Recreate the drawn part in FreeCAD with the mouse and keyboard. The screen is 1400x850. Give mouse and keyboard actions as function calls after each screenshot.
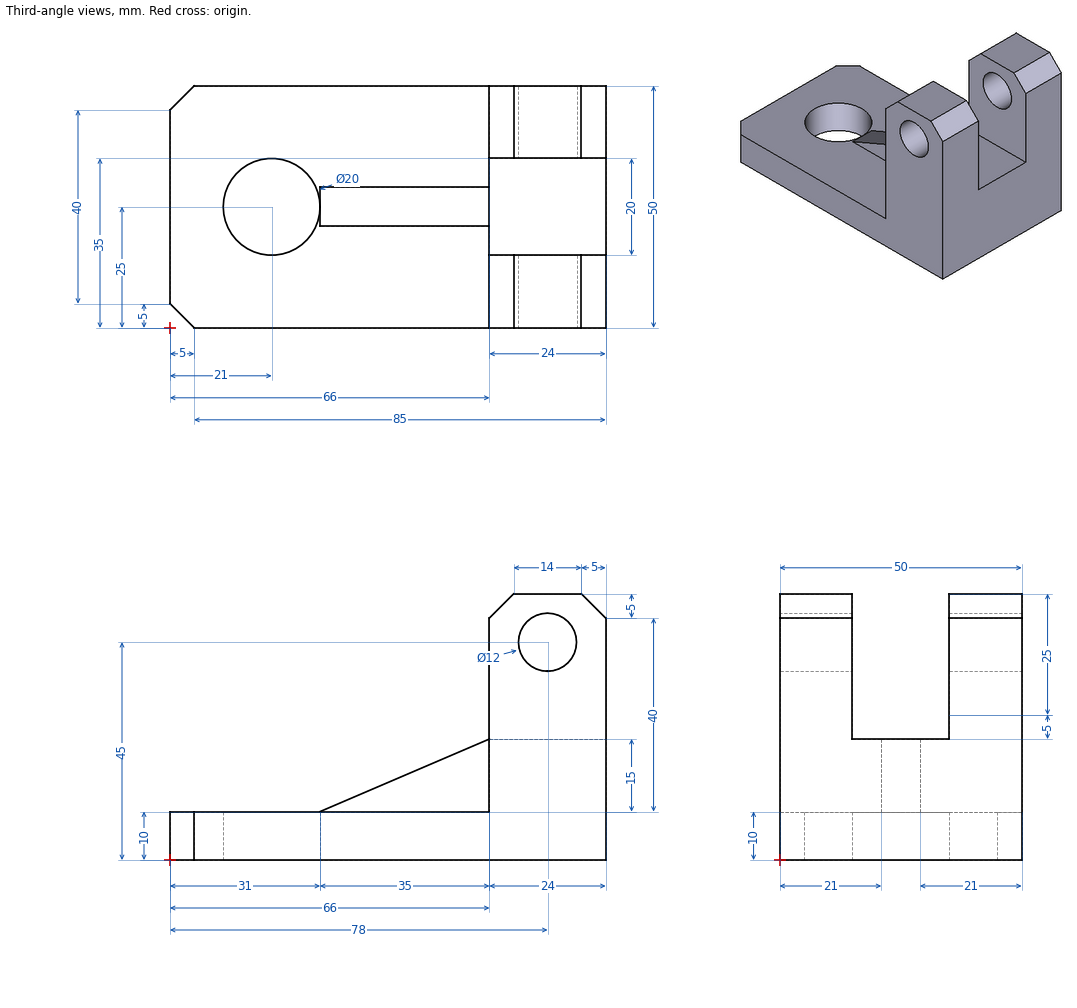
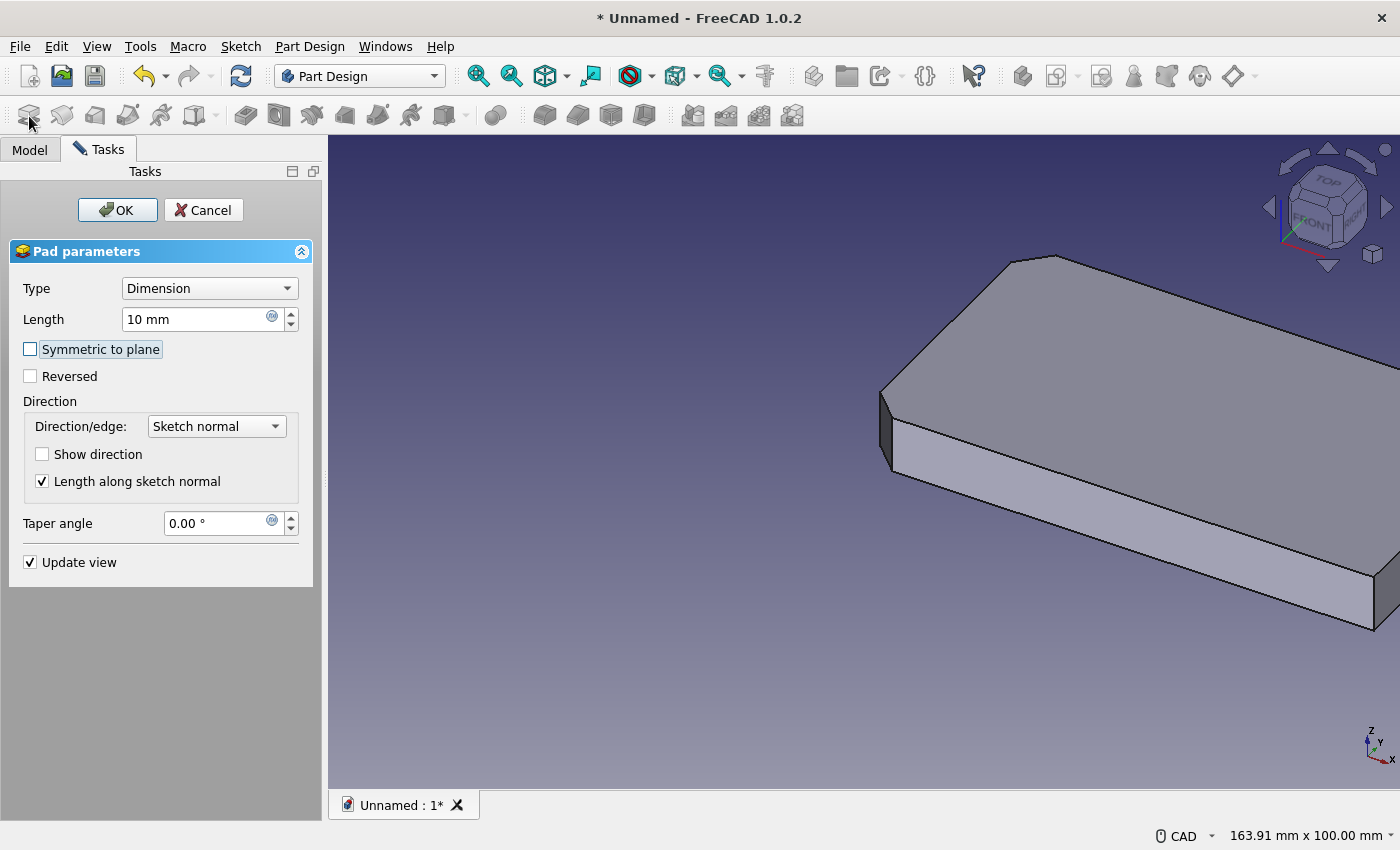
click(118, 210)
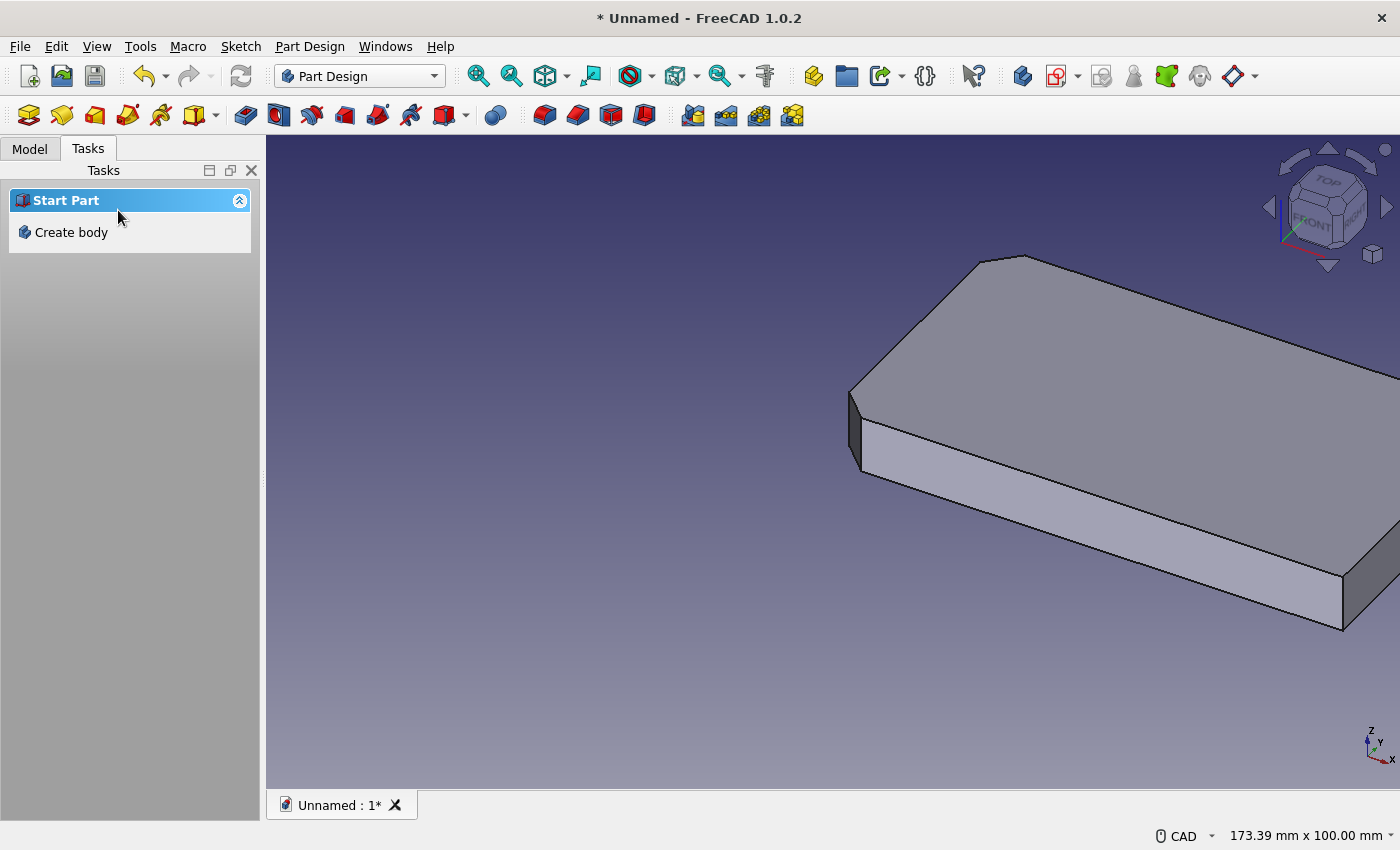
click(479, 76)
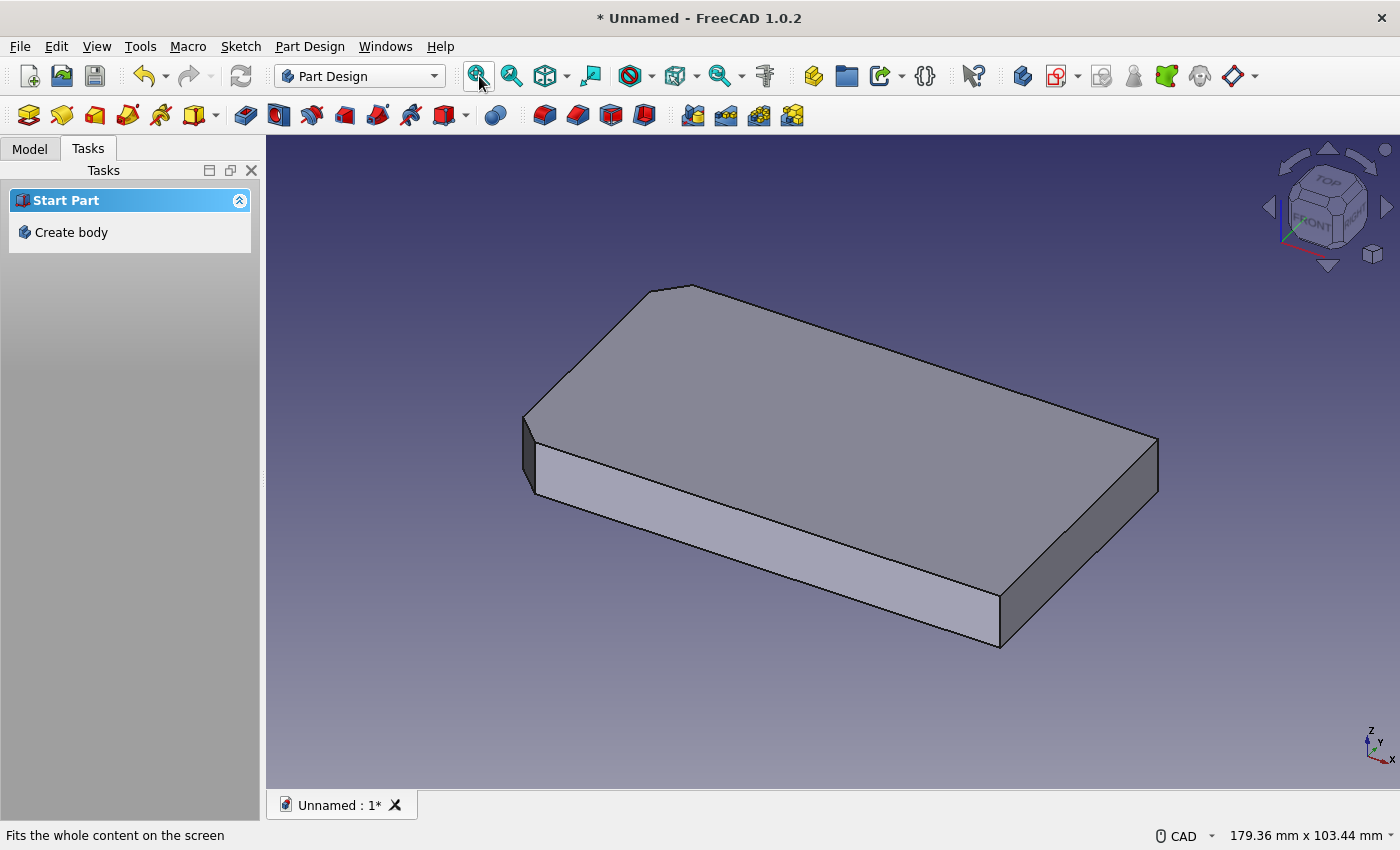
click(967, 610)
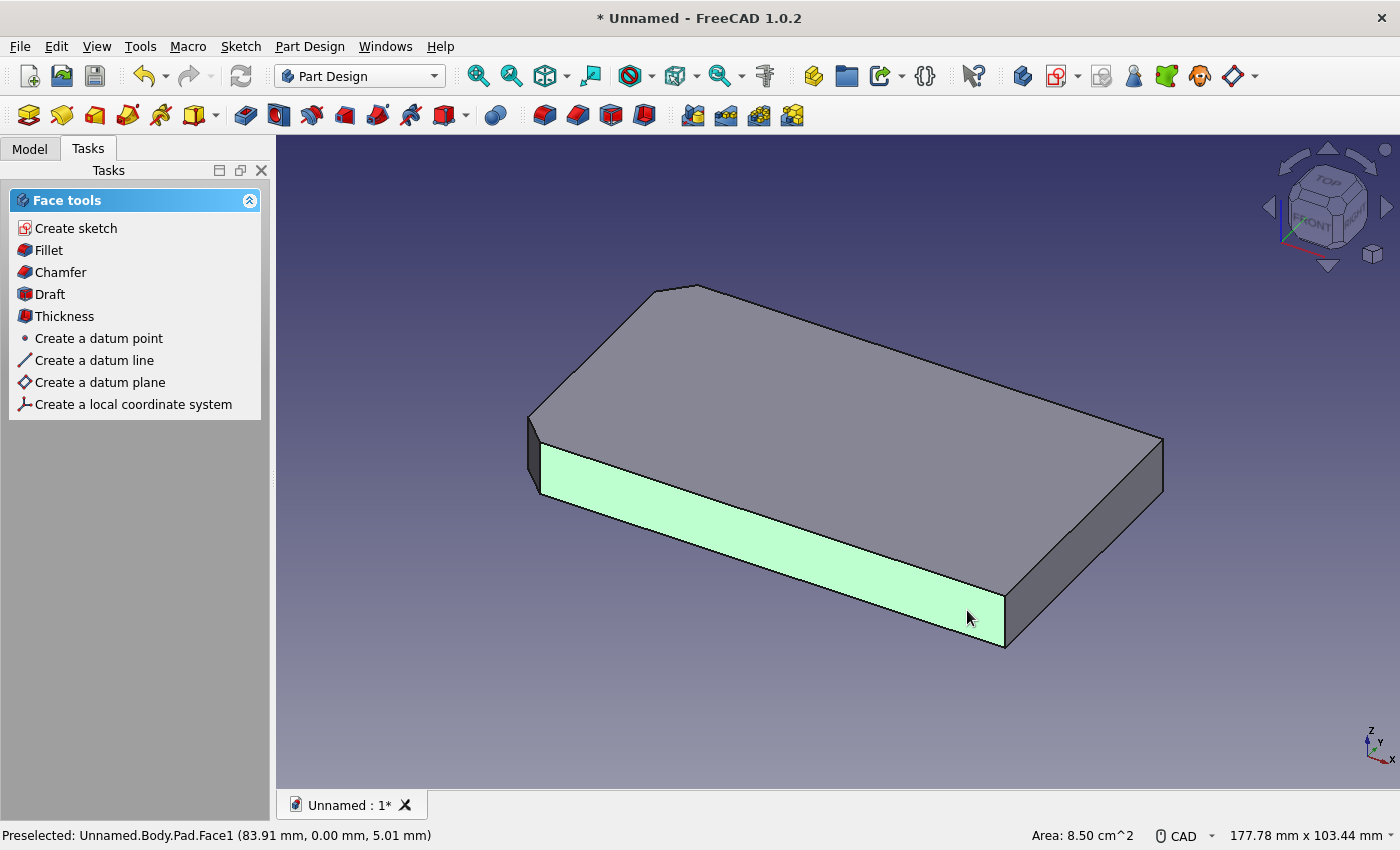
click(1056, 76)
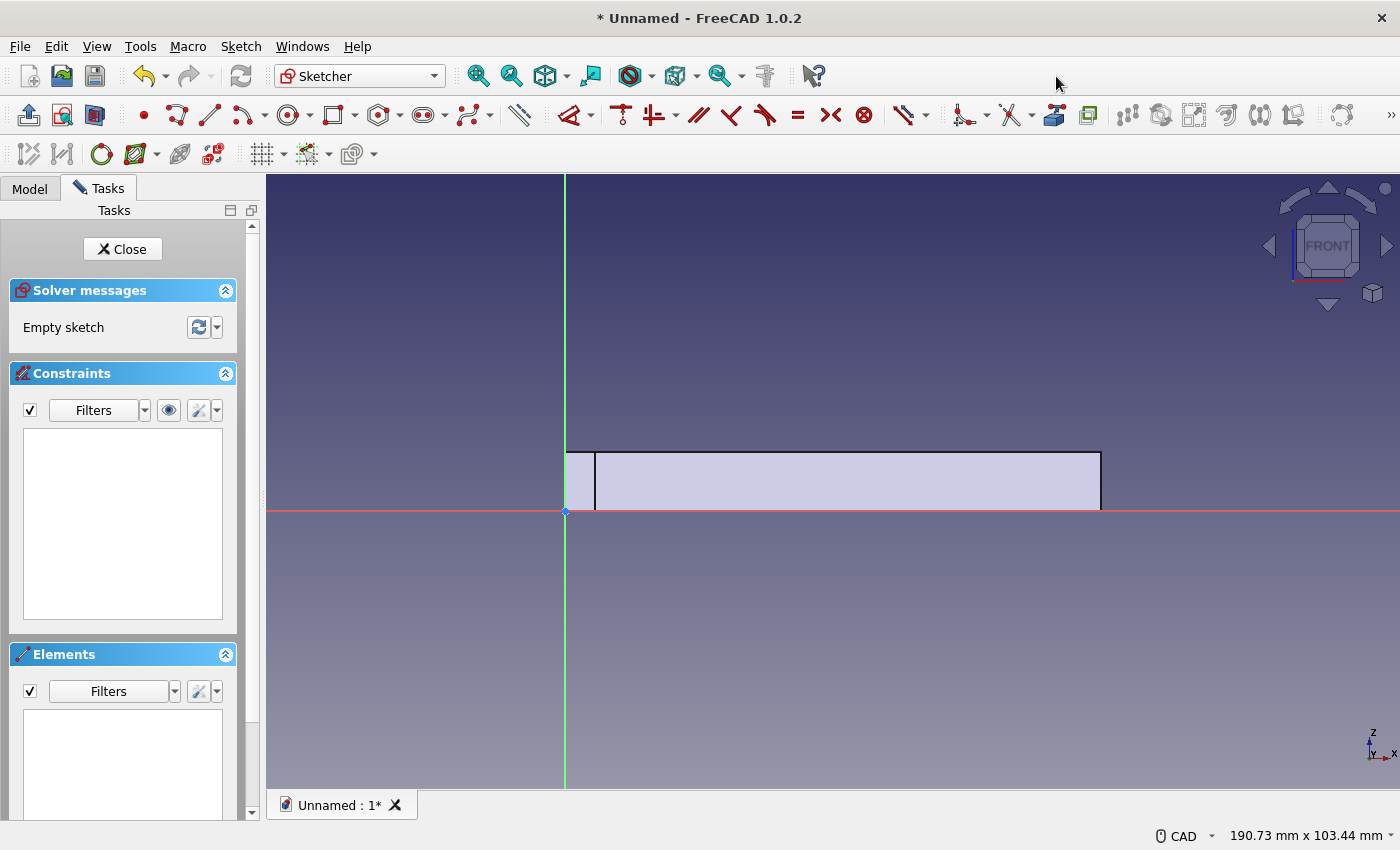
scroll(455, 761, down, 1)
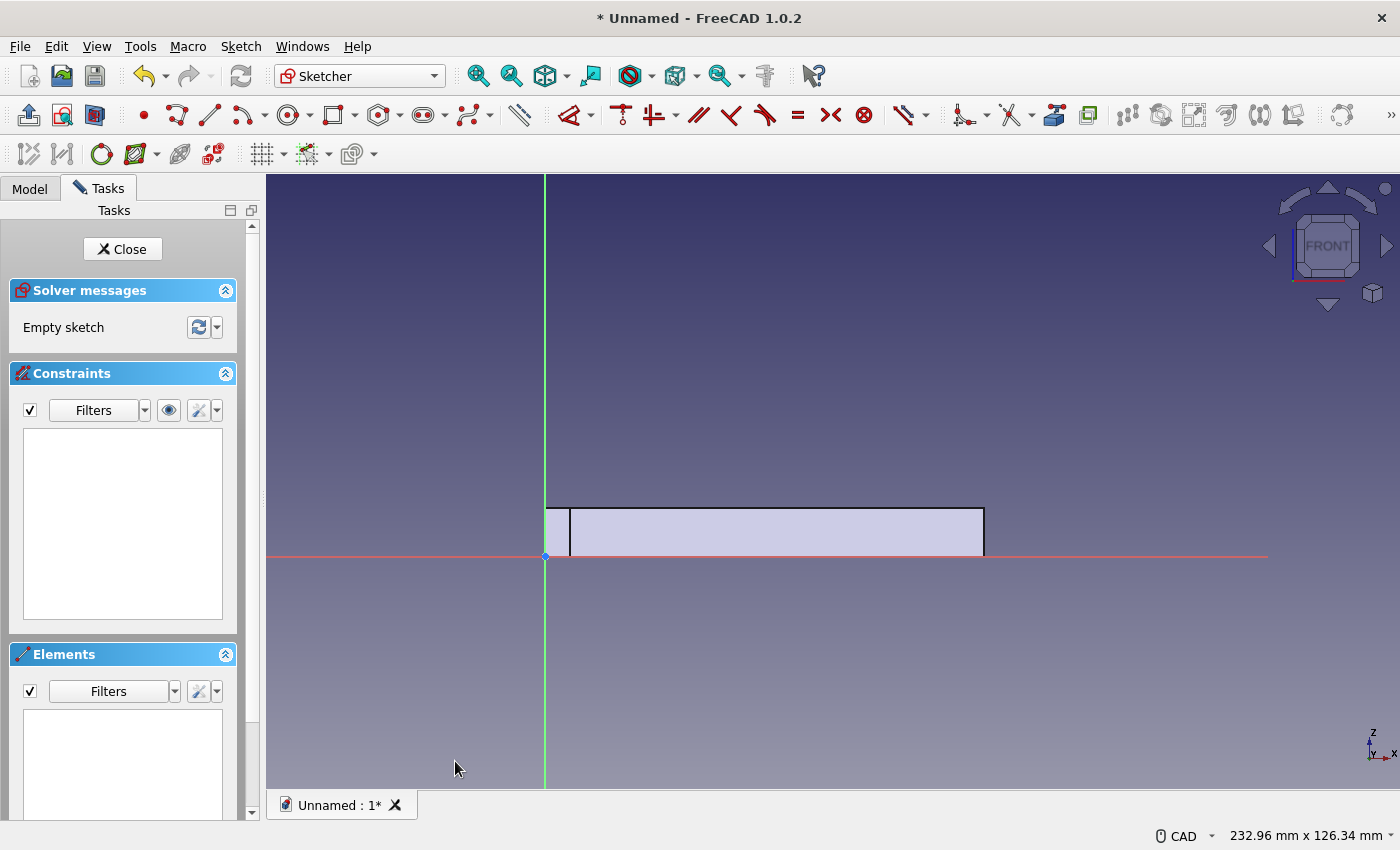
scroll(765, 303, up, 2)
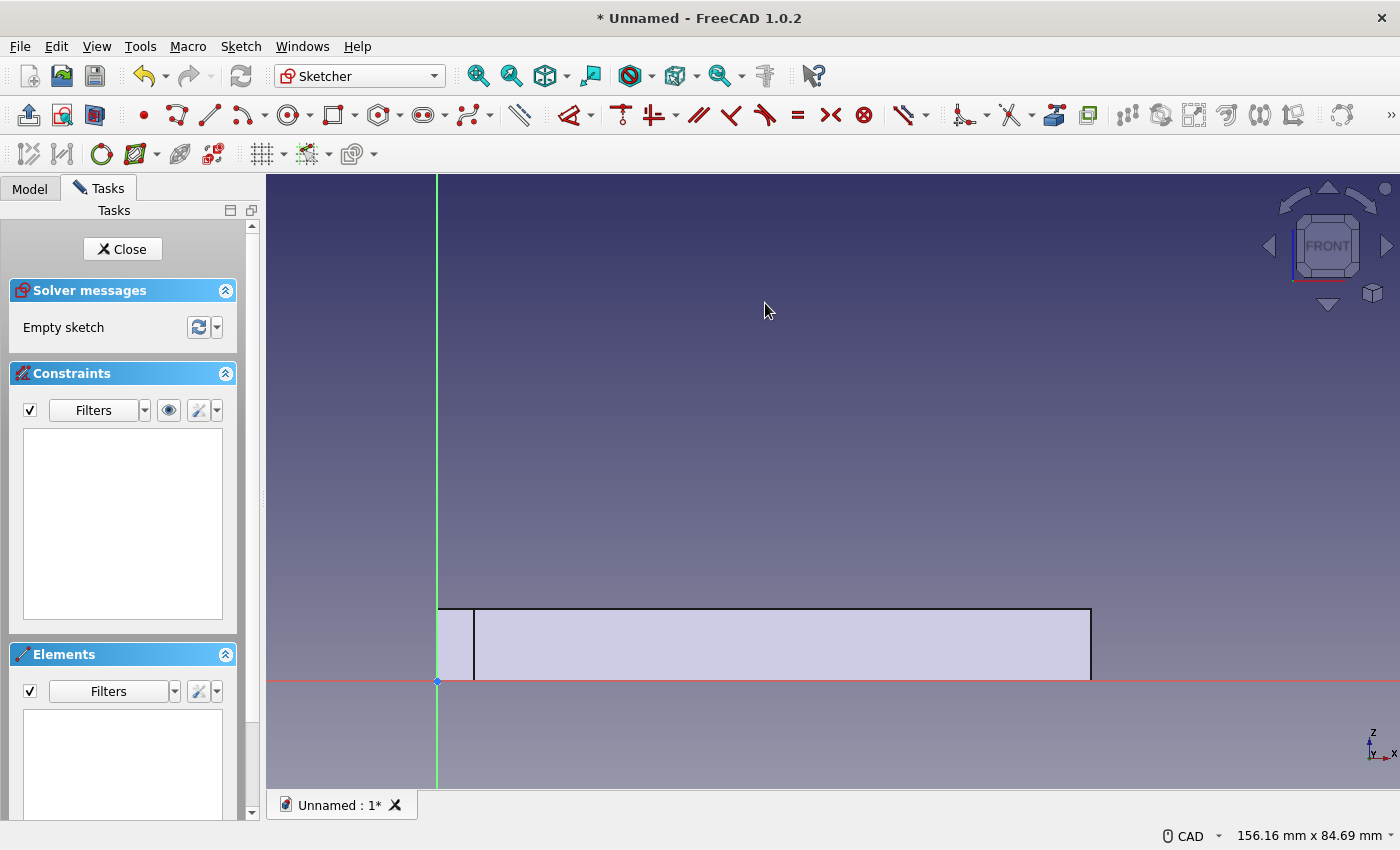
click(177, 116)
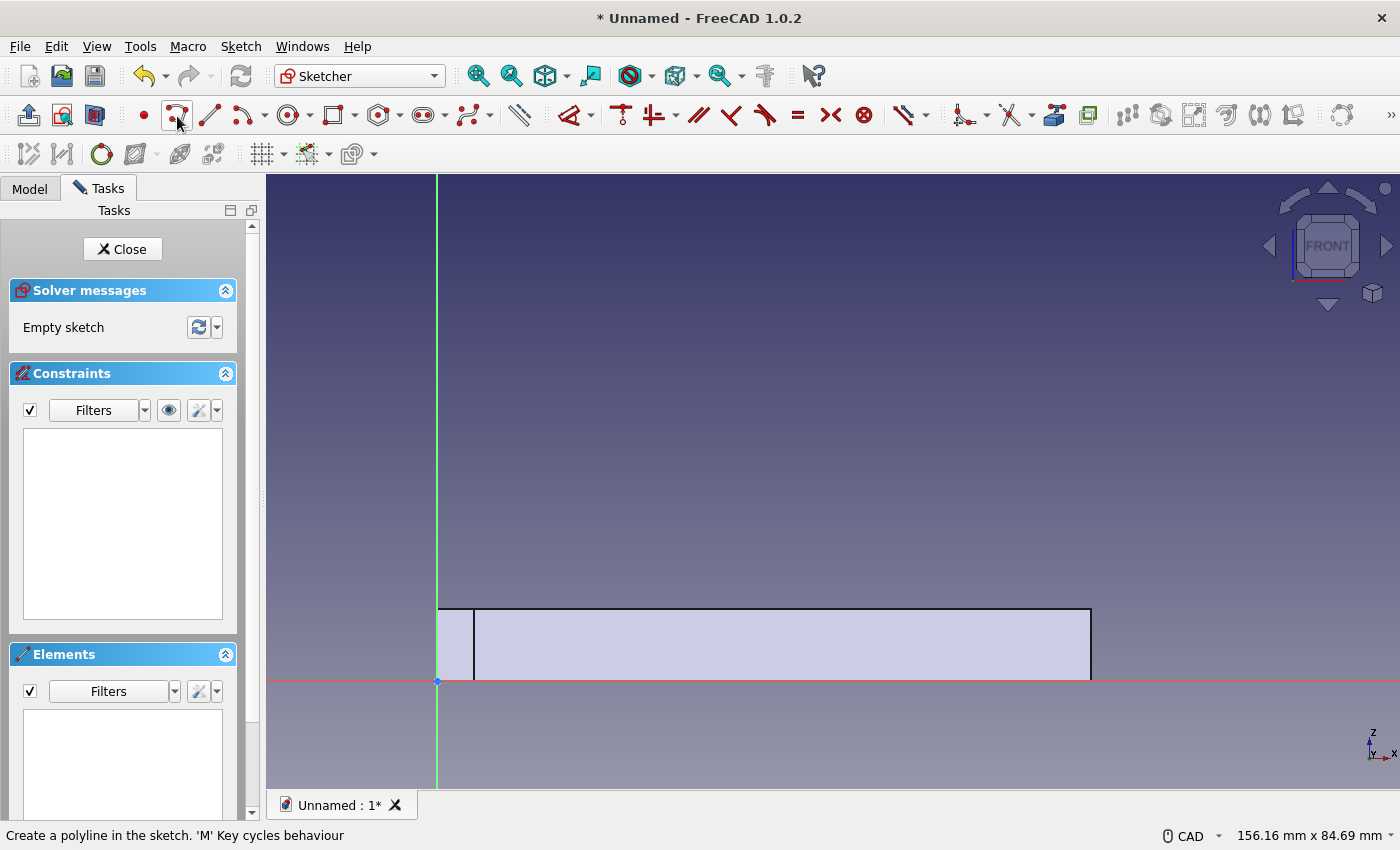
click(917, 609)
click(1091, 609)
click(1091, 318)
click(1055, 282)
click(953, 282)
click(917, 318)
click(917, 610)
key(Escape)
key(Escape)